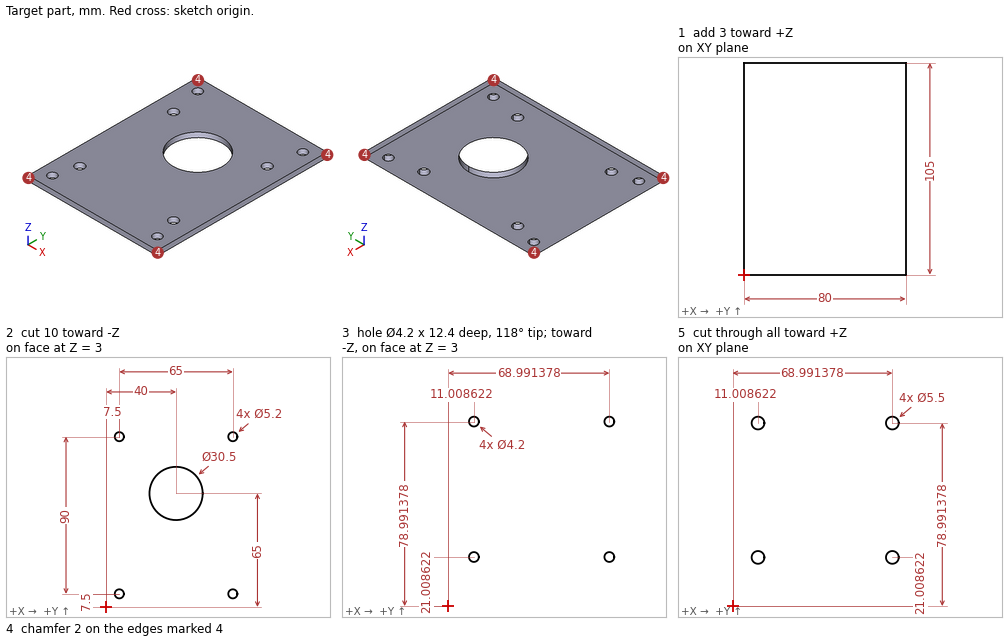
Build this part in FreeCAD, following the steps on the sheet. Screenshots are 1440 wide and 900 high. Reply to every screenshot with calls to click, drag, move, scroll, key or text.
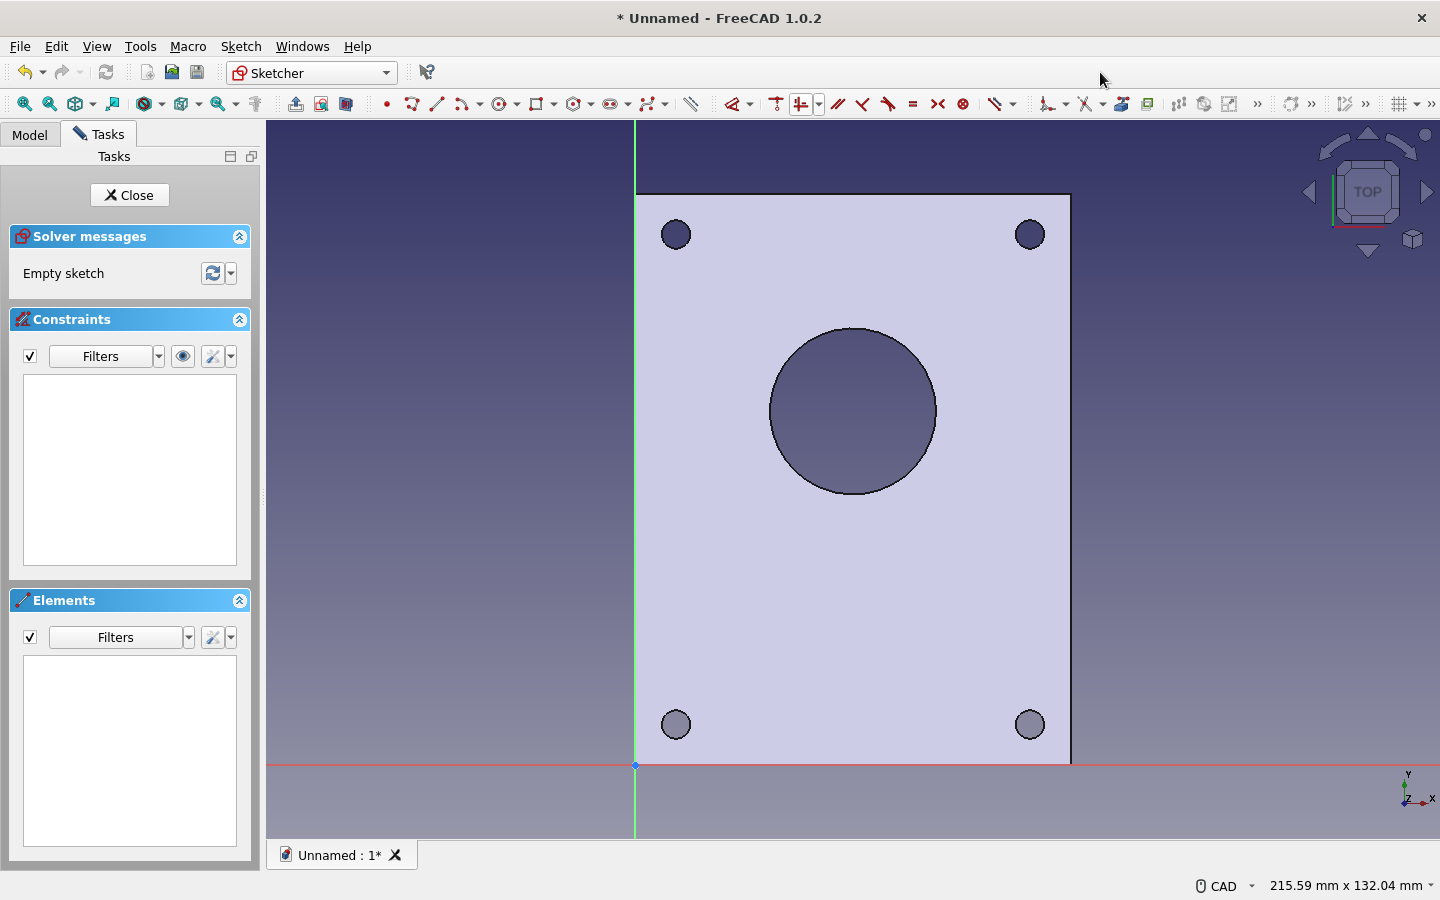
click(498, 104)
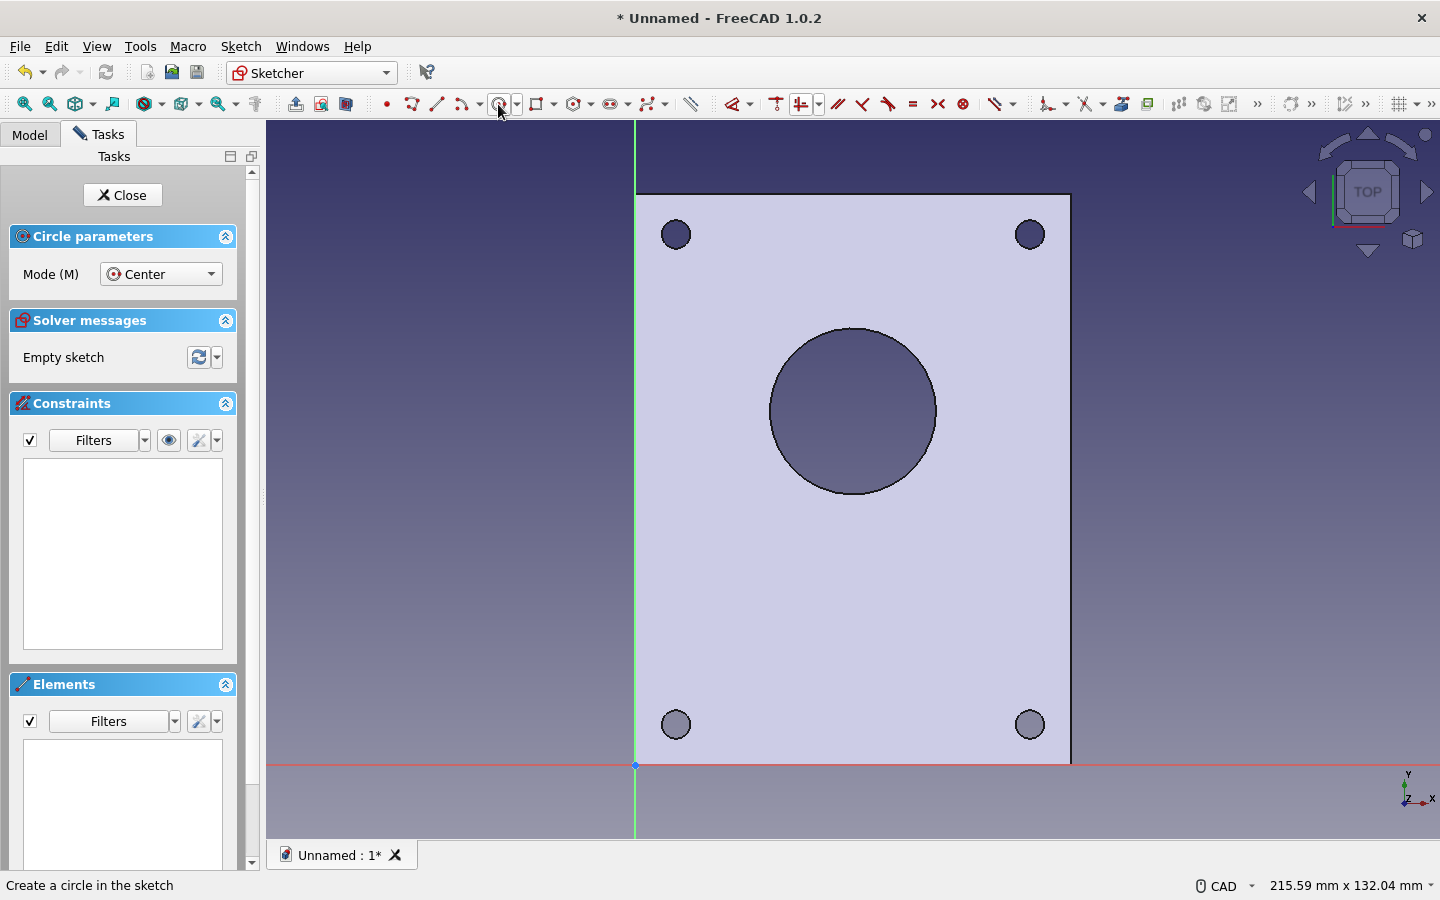
scroll(695, 335, up, 4)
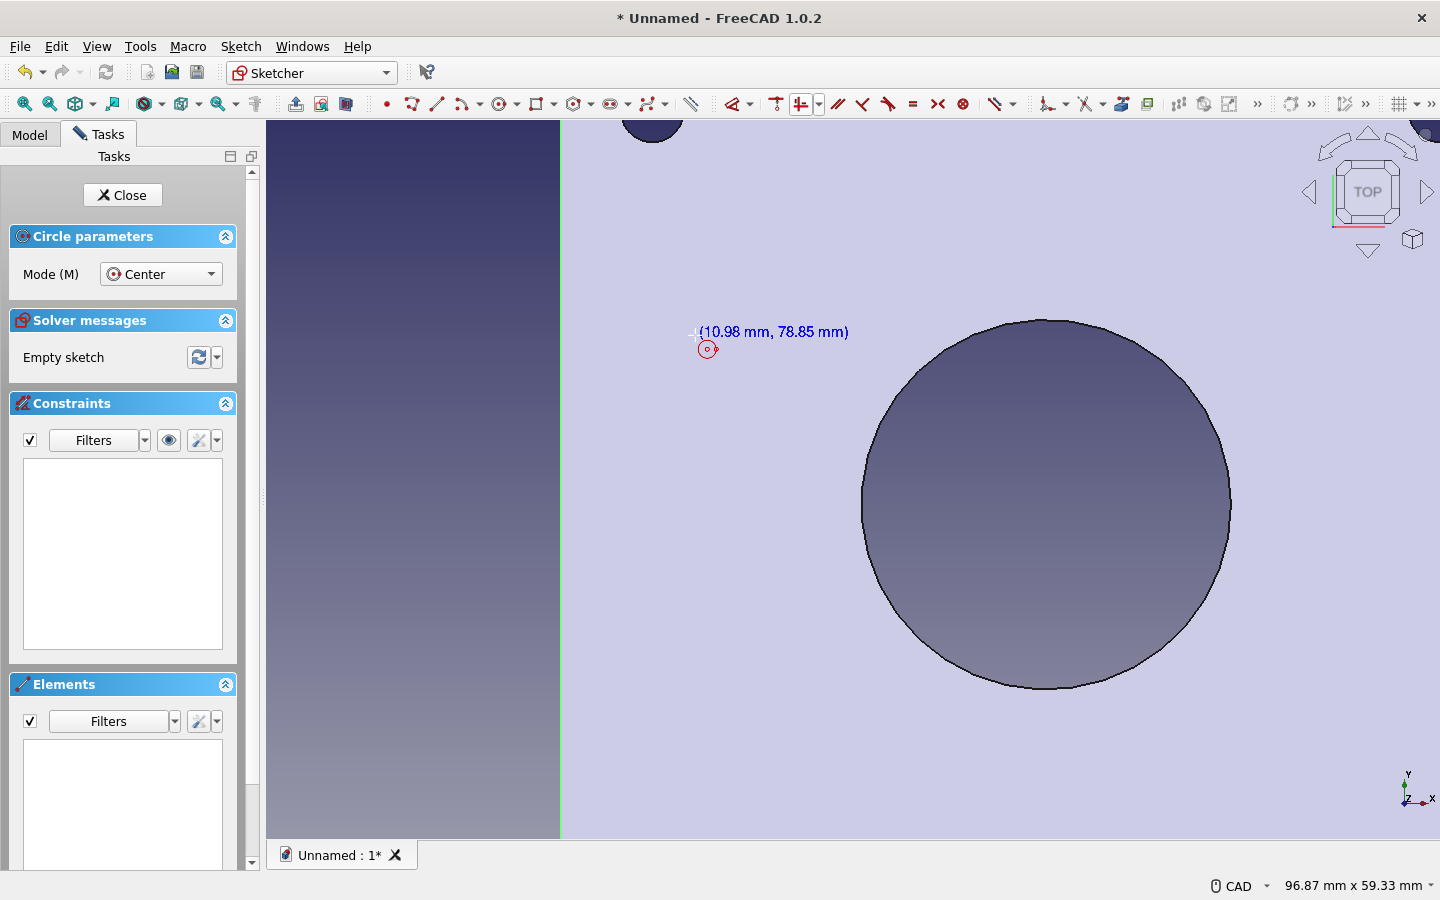
click(695, 335)
click(713, 317)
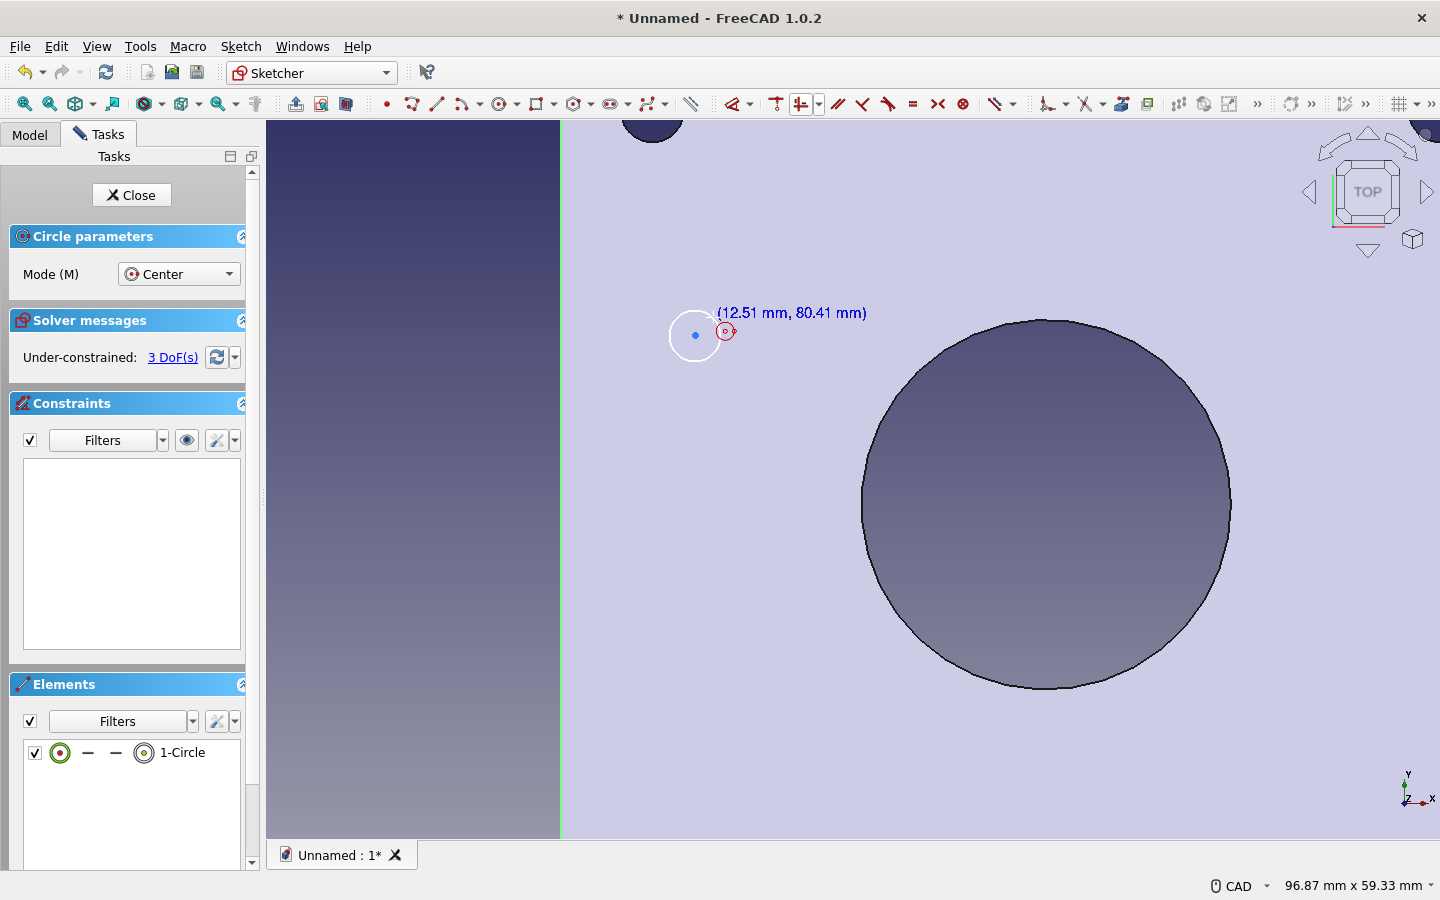
scroll(615, 217, down, 4)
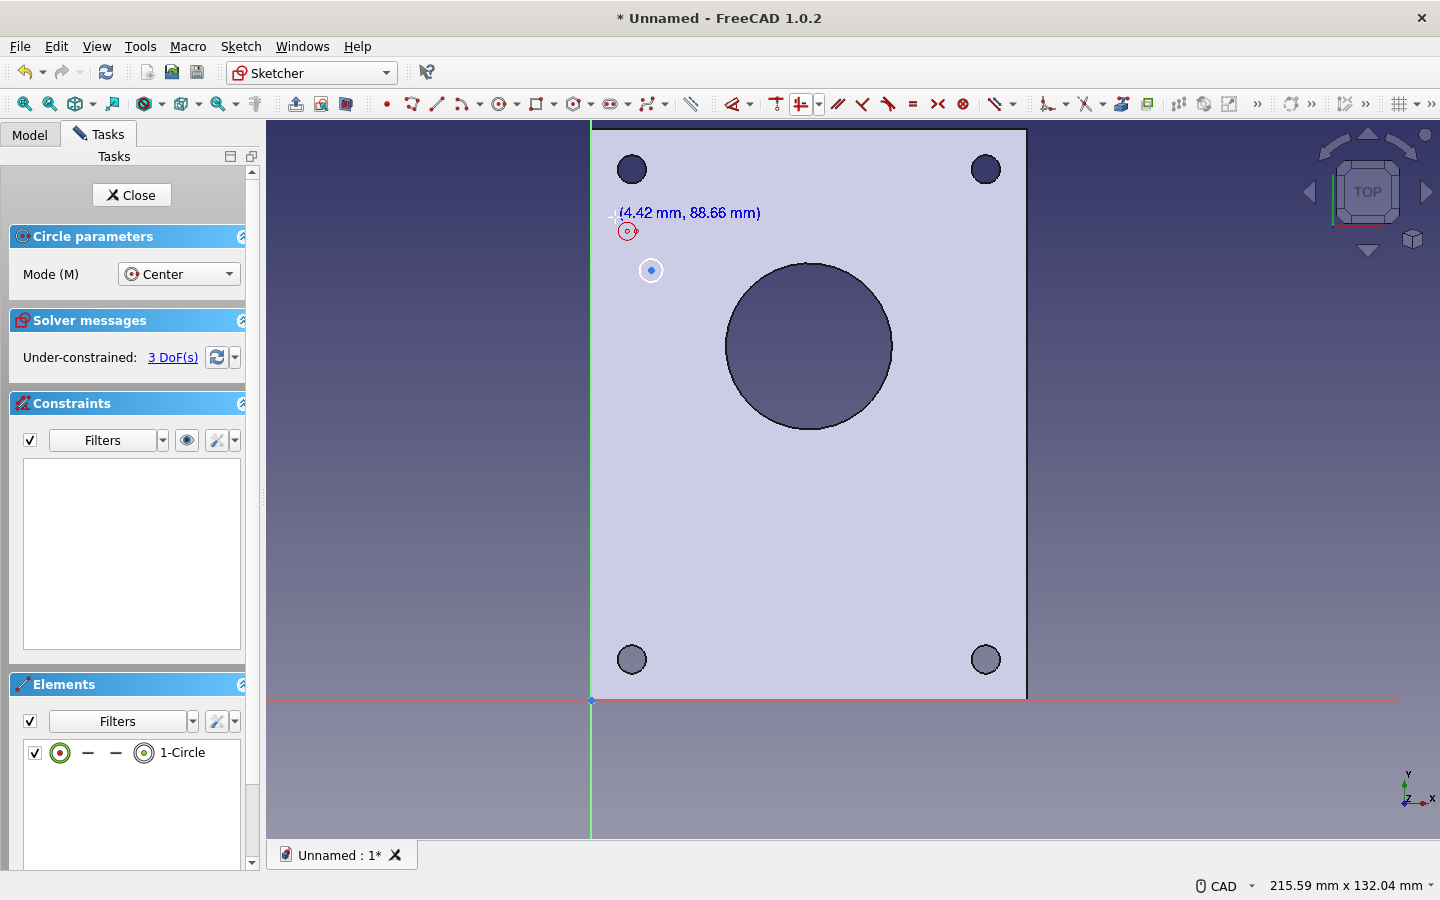
scroll(967, 270, up, 4)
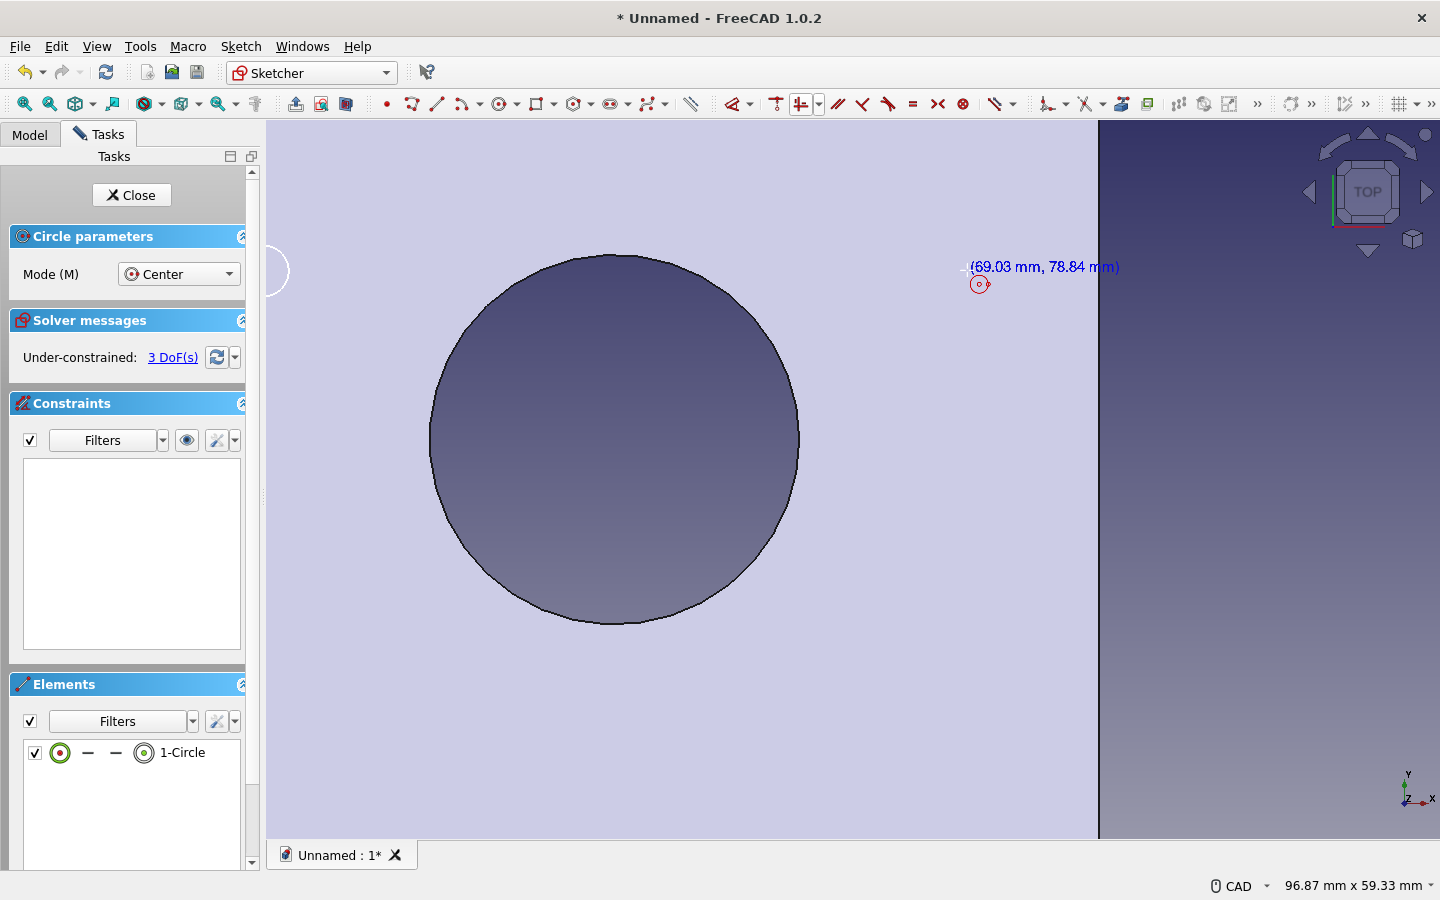
click(966, 270)
click(984, 252)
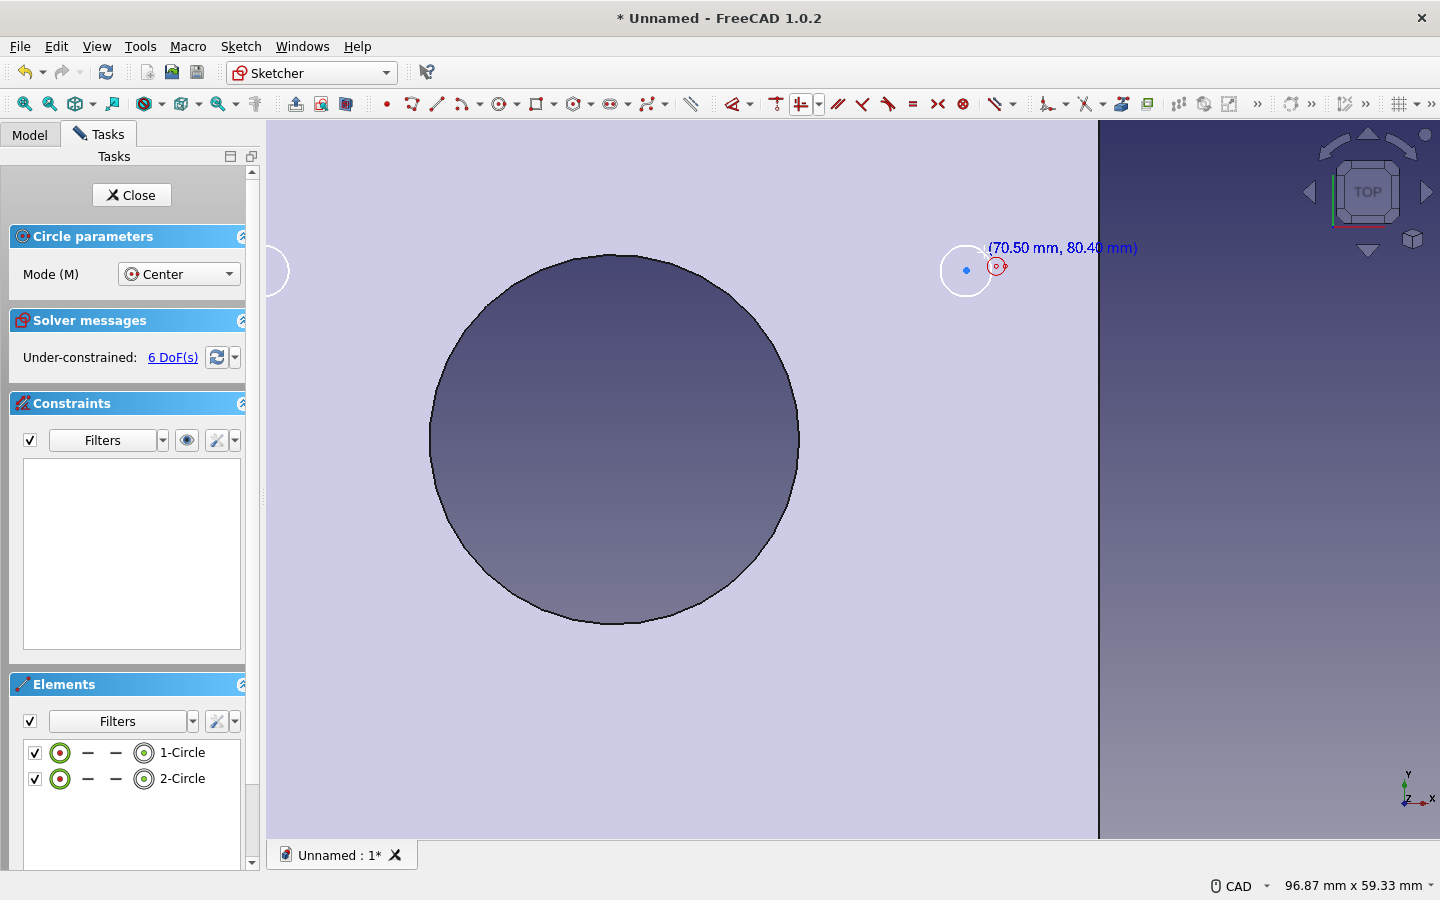
scroll(967, 270, down, 4)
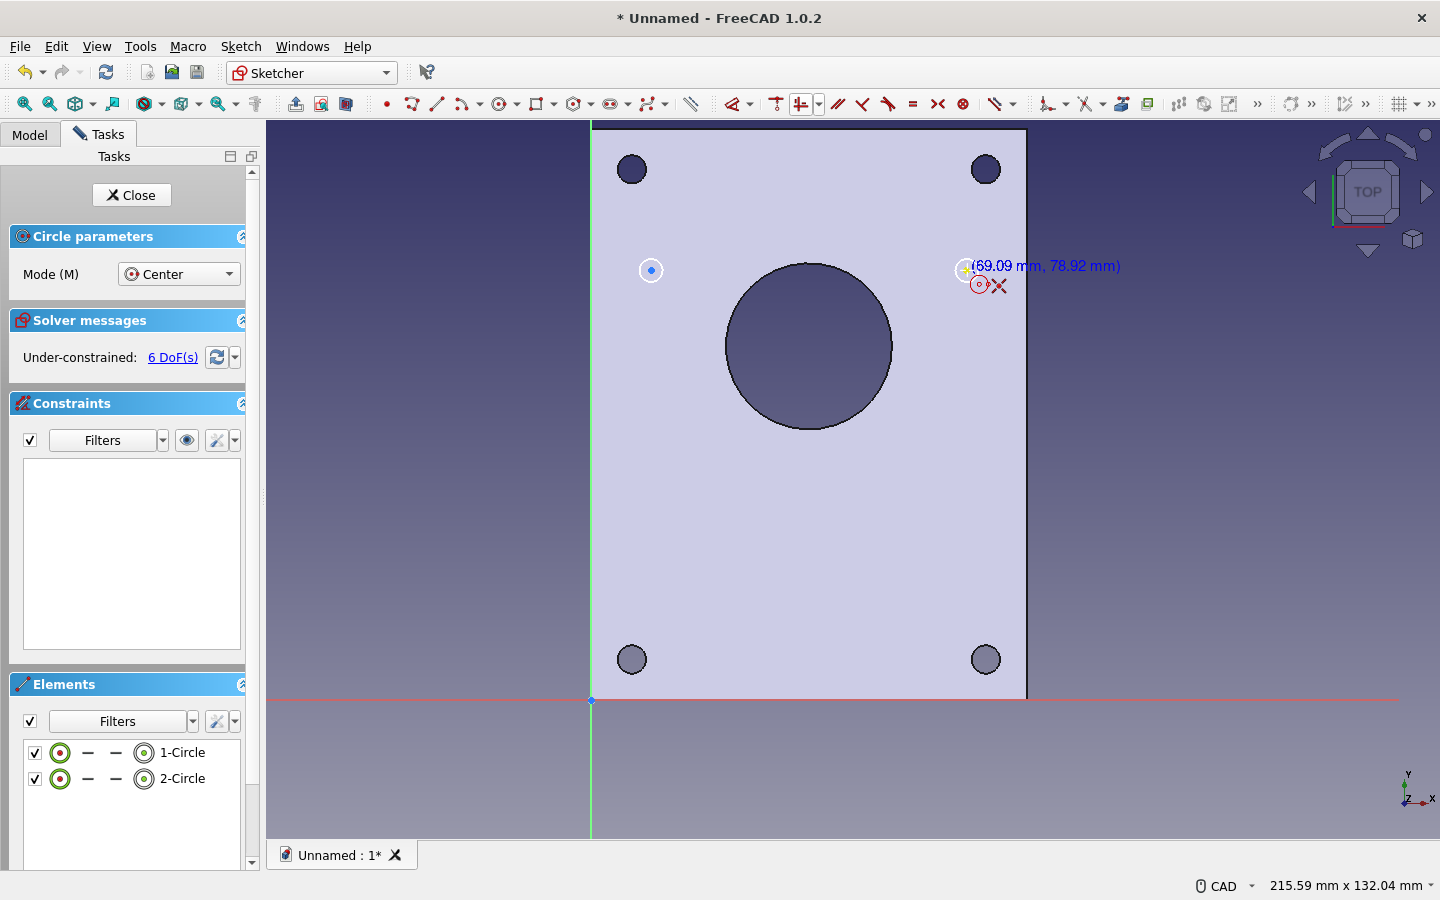
scroll(651, 586, up, 4)